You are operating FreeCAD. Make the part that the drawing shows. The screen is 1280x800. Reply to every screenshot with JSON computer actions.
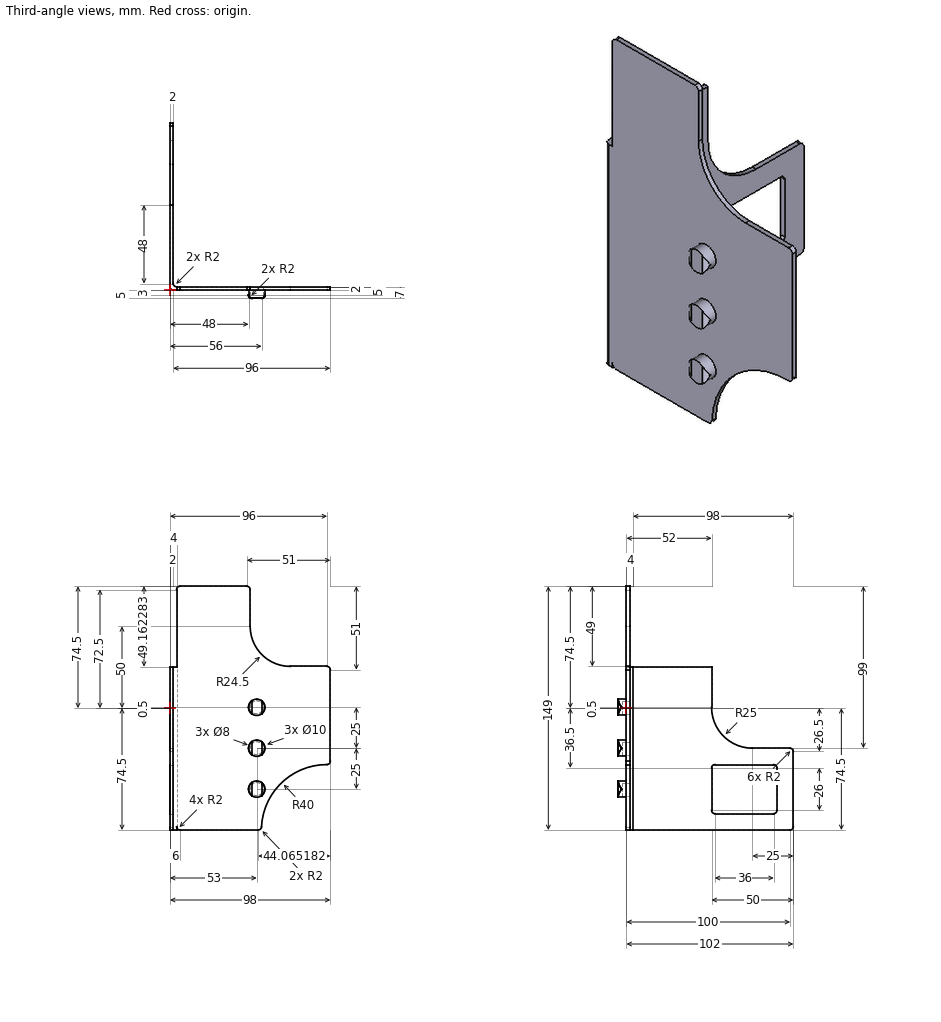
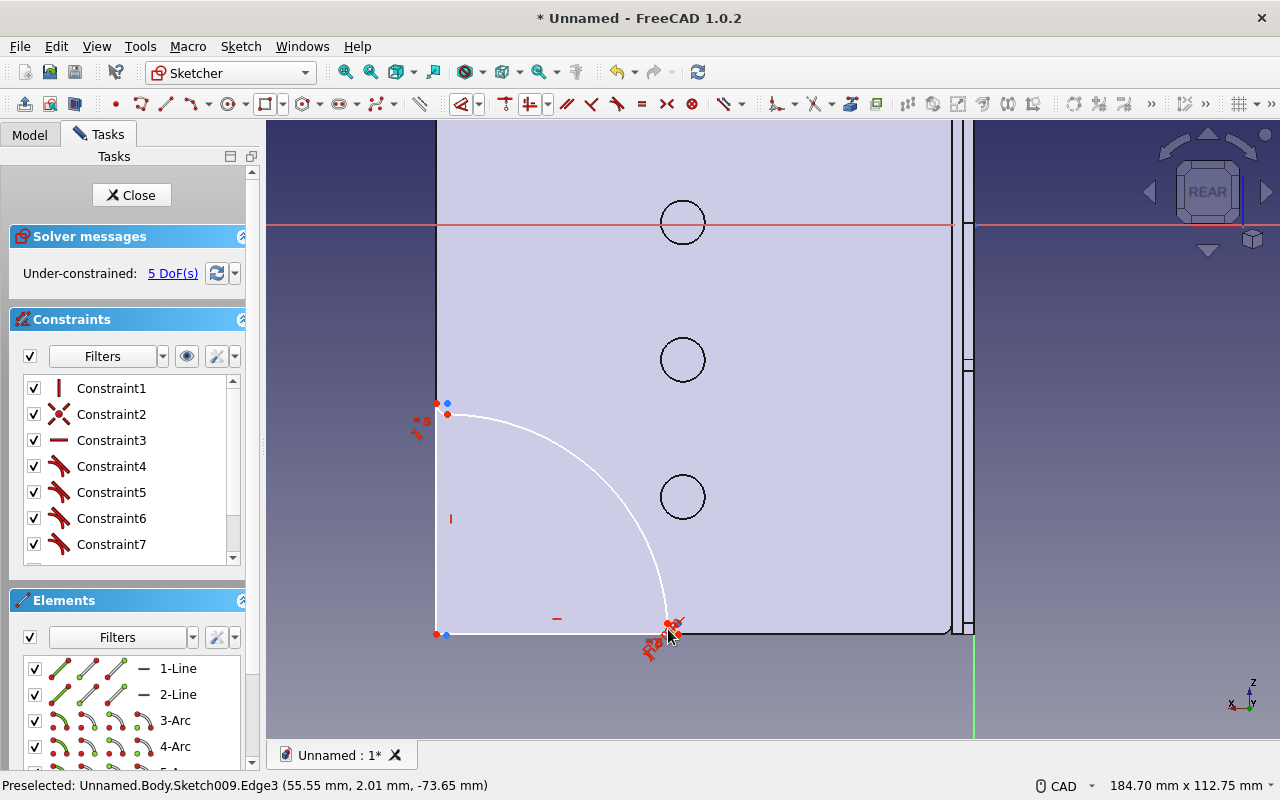
{"action": "left_click", "coordinate": [640, 528]}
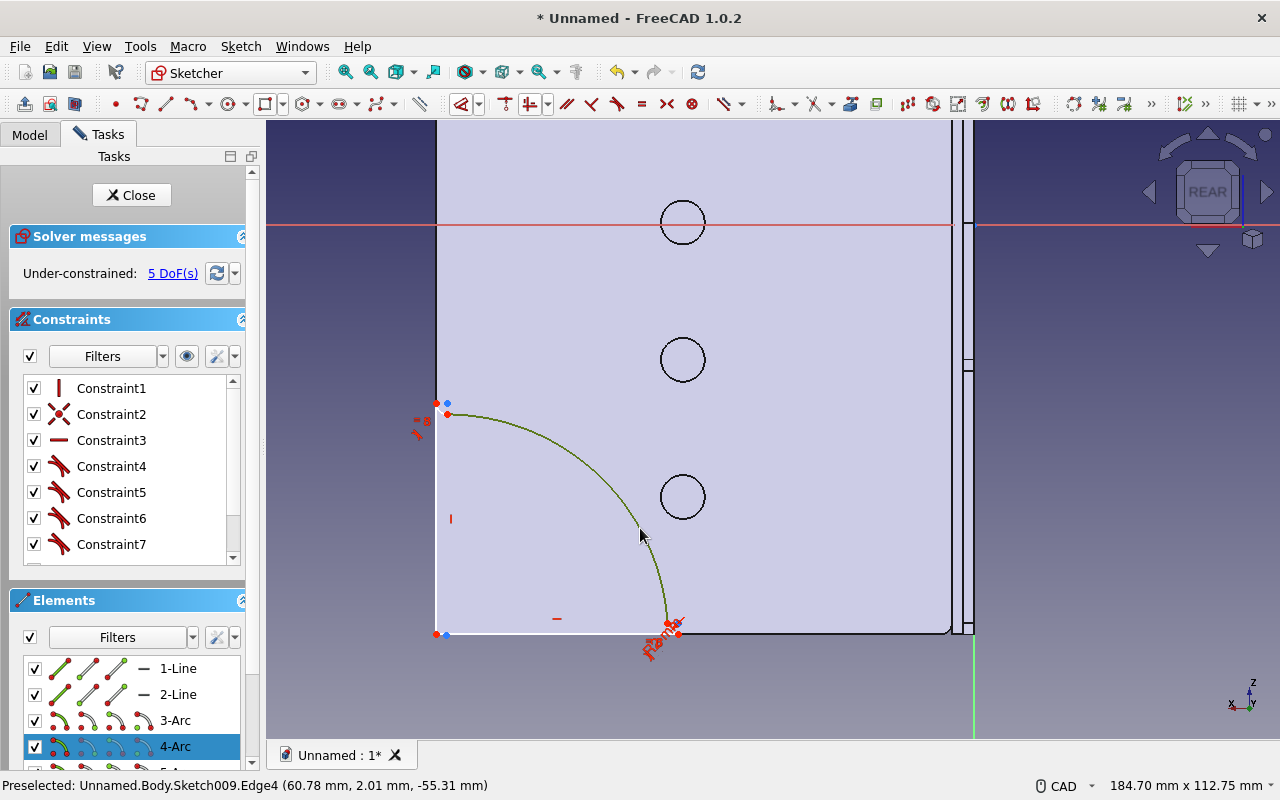
{"action": "key", "text": "k r"}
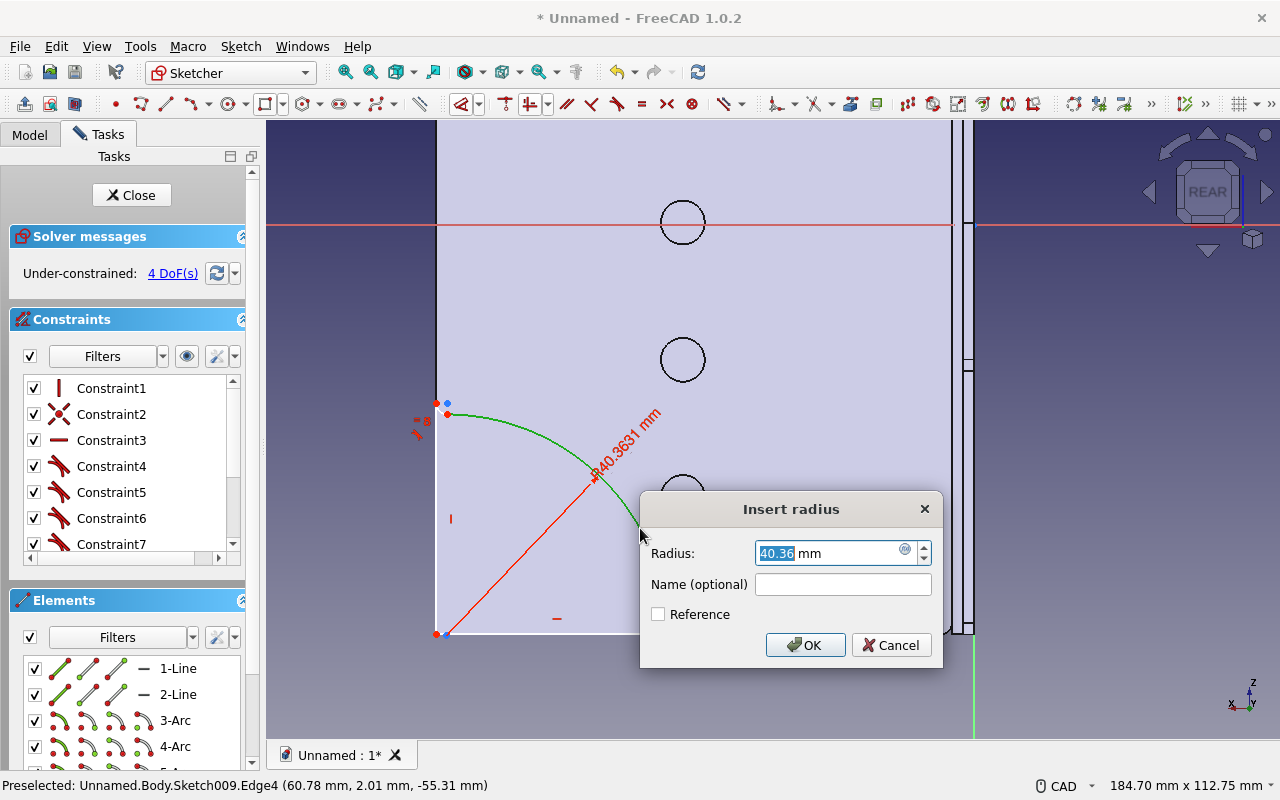
{"action": "type", "text": "40"}
{"action": "key", "text": "Return"}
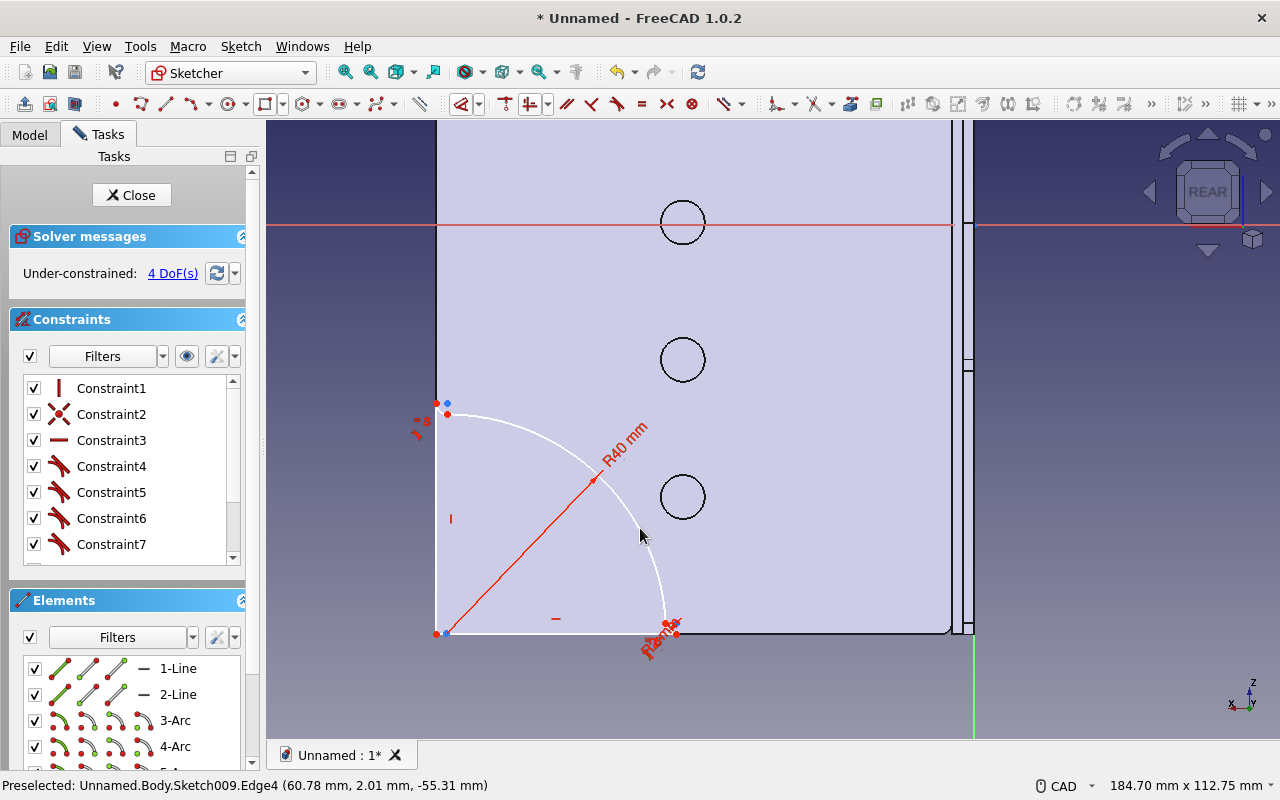
{"action": "left_click", "coordinate": [436, 403]}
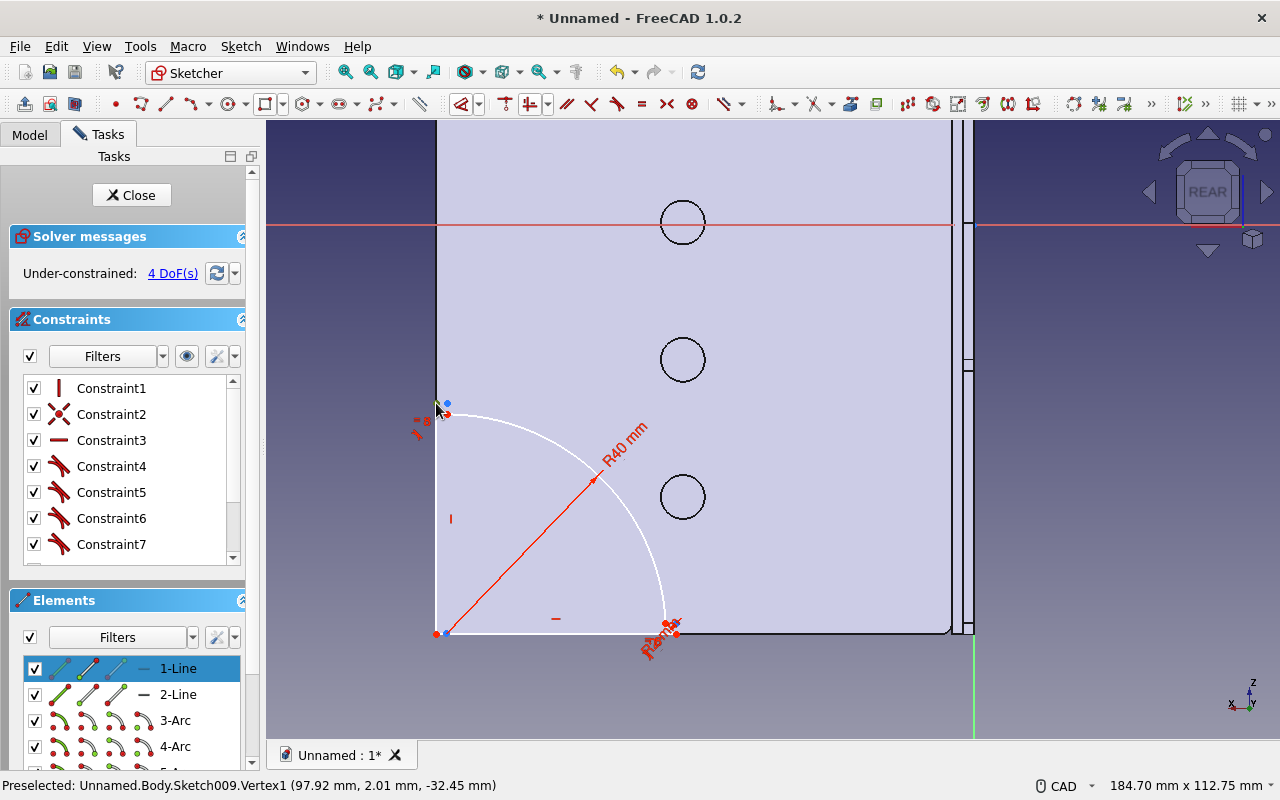
{"action": "key", "text": "l"}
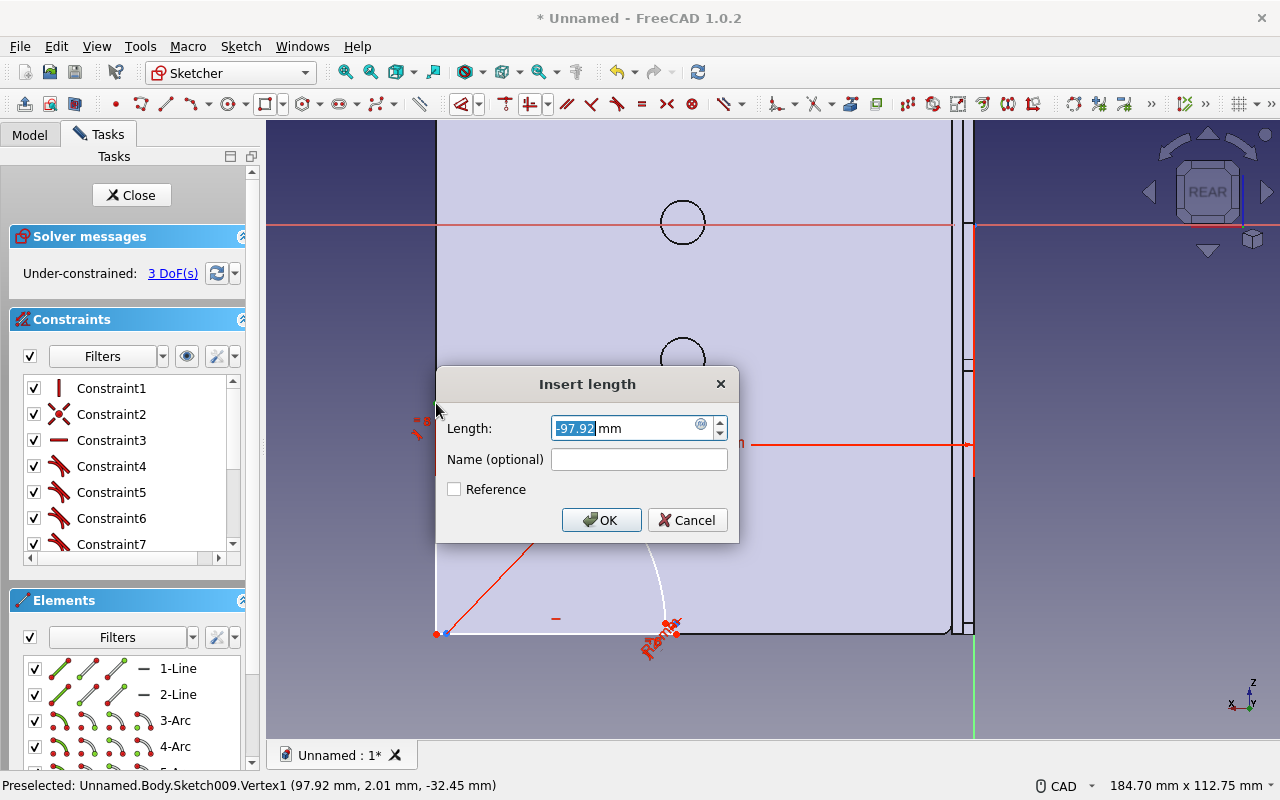
{"action": "type", "text": "-98"}
{"action": "key", "text": "Return"}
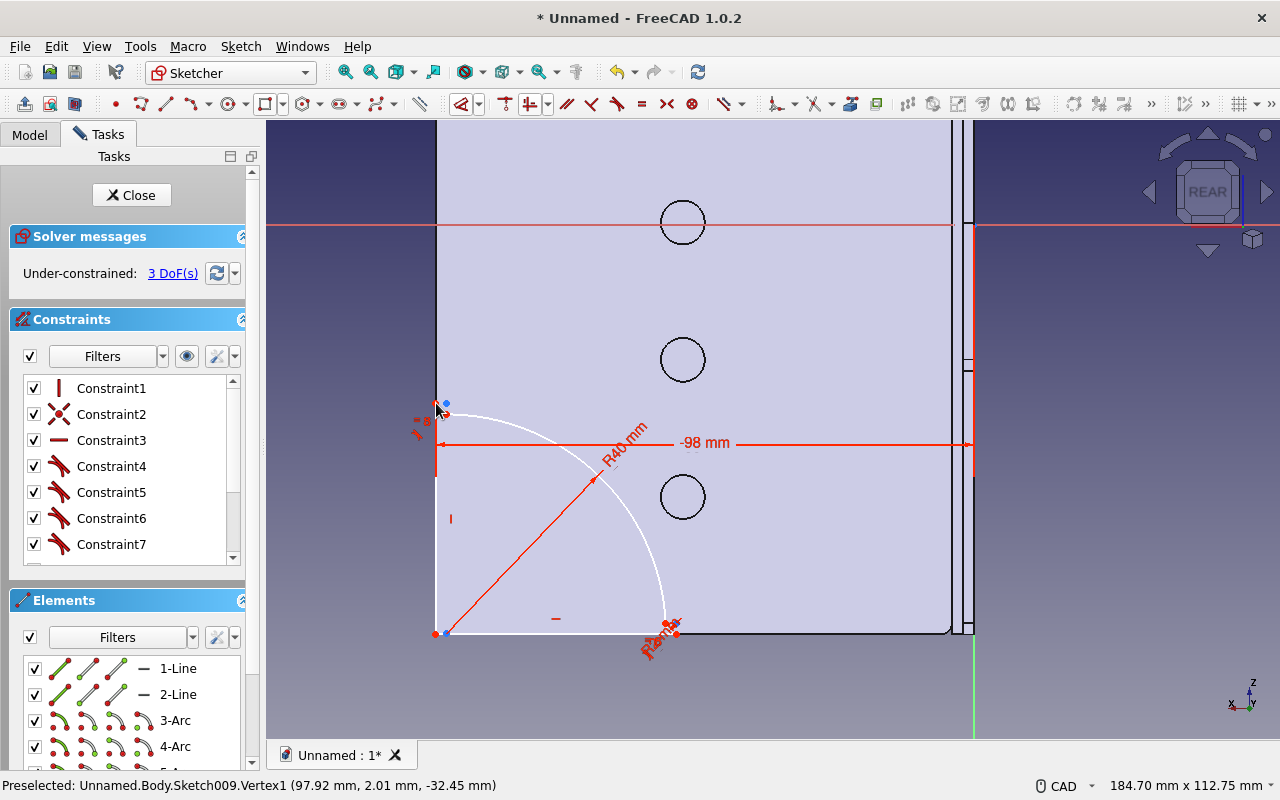
{"action": "left_click", "coordinate": [436, 634]}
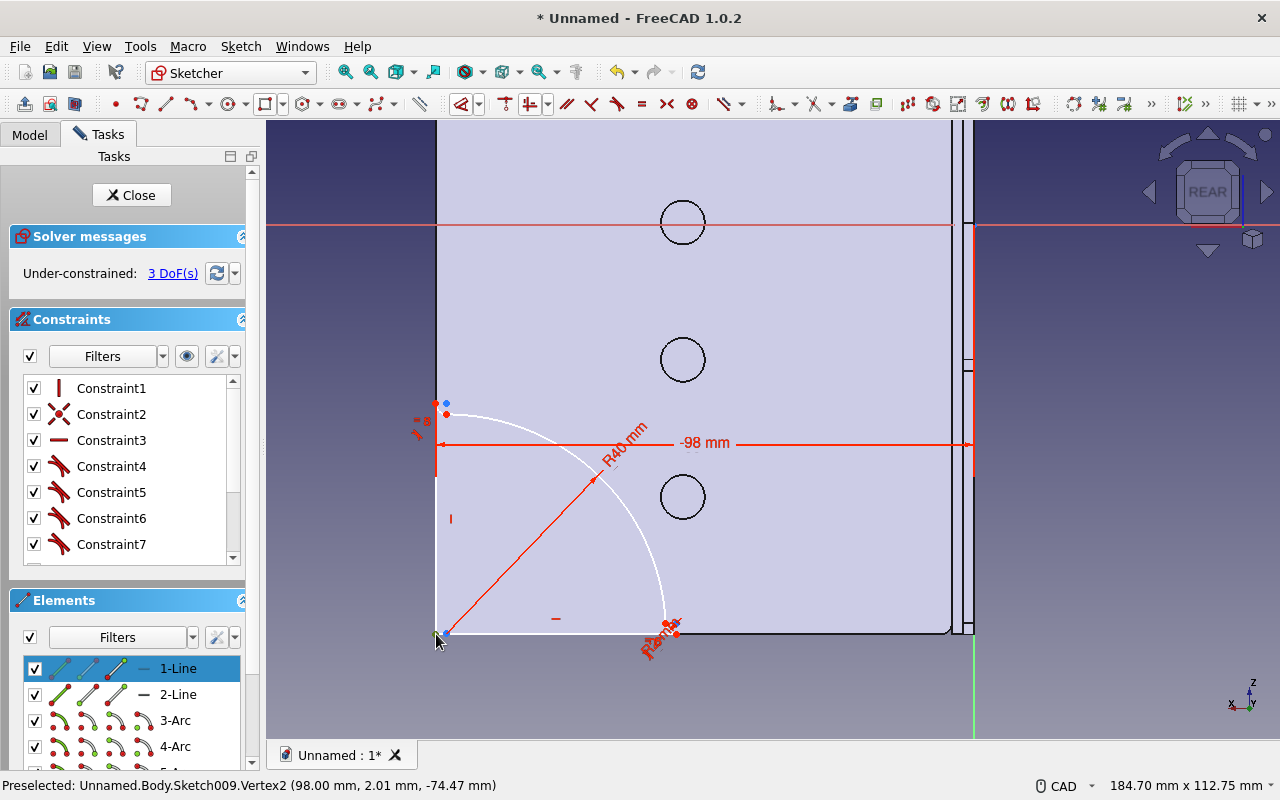
{"action": "key", "text": "i"}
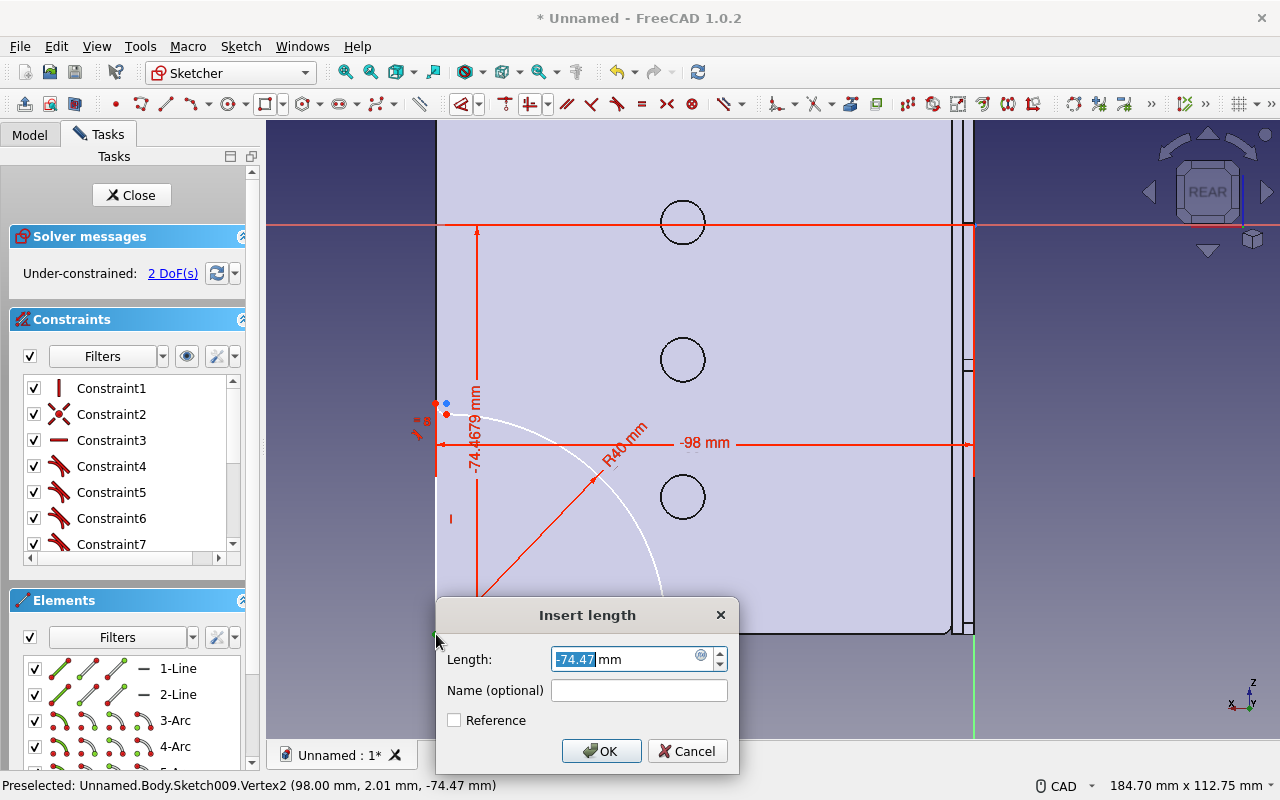
{"action": "type", "text": "-74.5"}
{"action": "key", "text": "Return"}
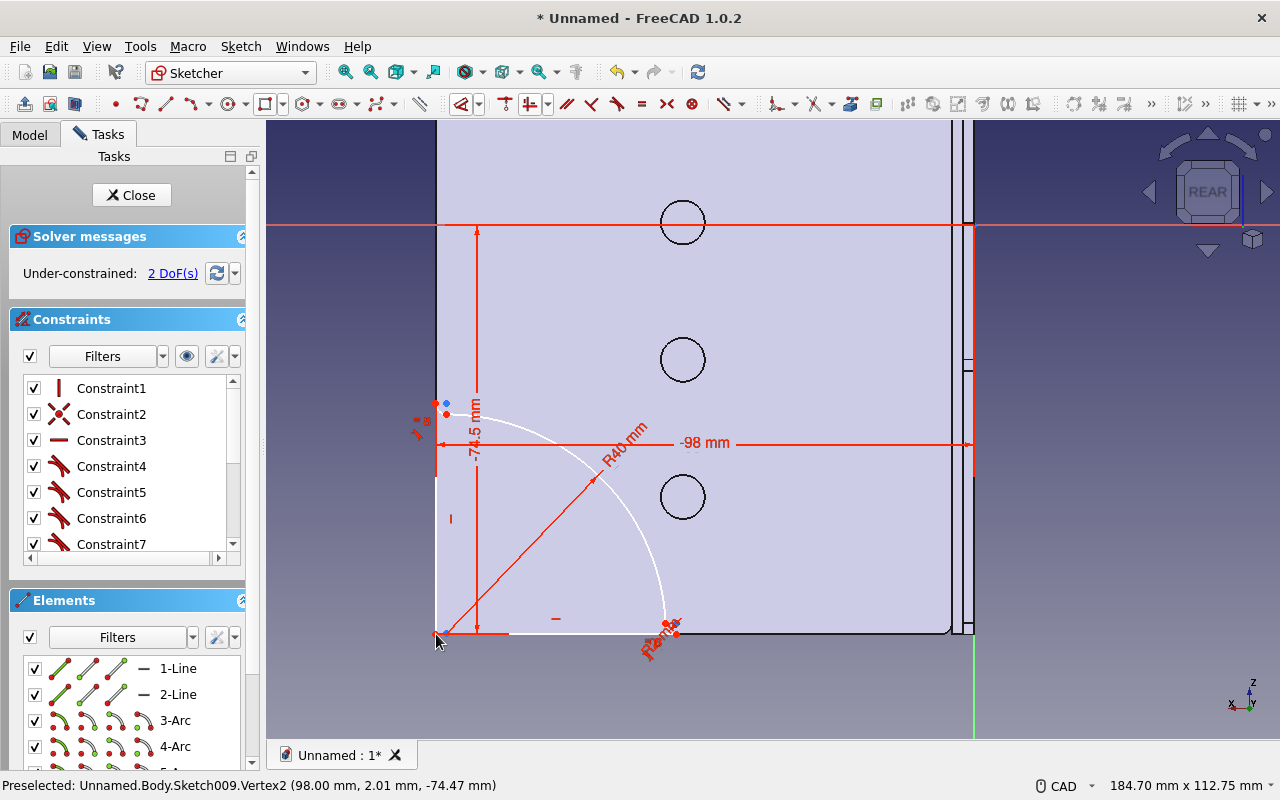
{"action": "left_click", "coordinate": [446, 634]}